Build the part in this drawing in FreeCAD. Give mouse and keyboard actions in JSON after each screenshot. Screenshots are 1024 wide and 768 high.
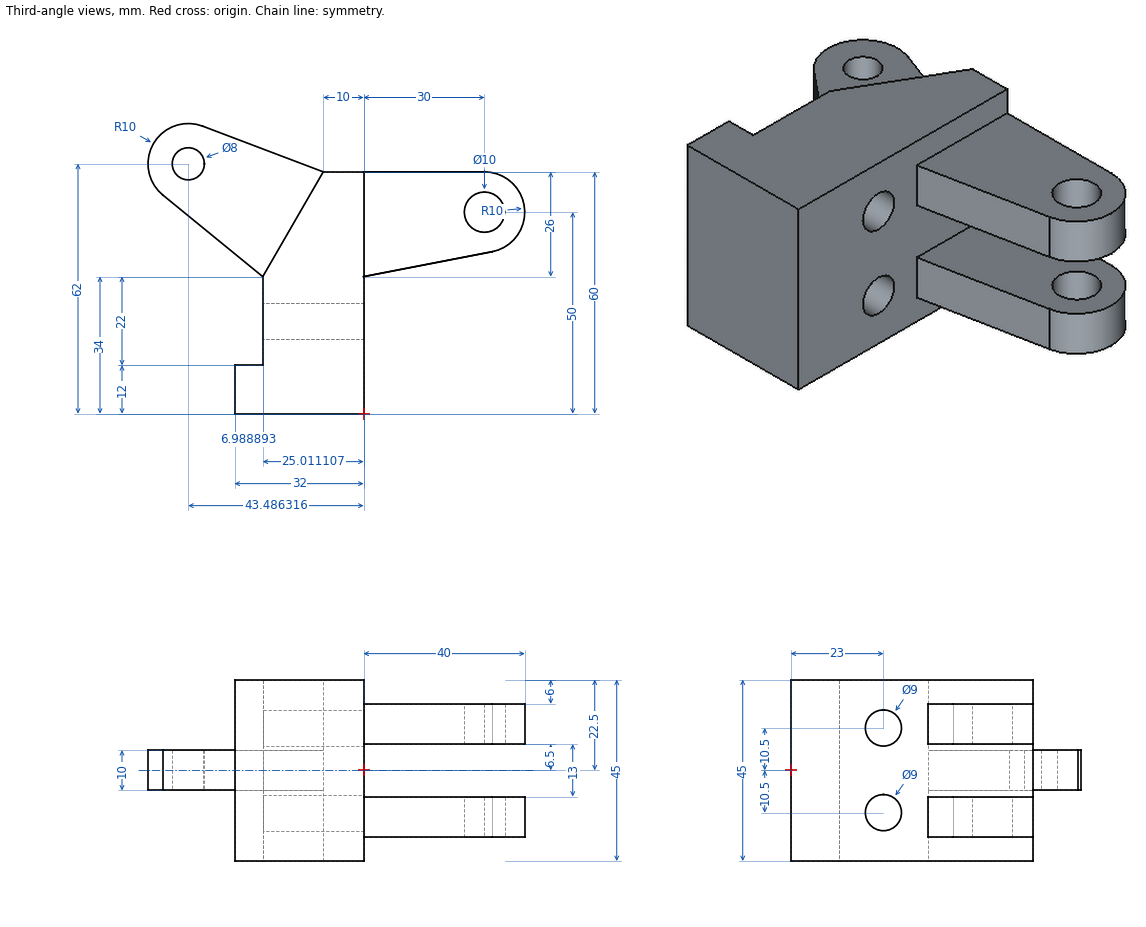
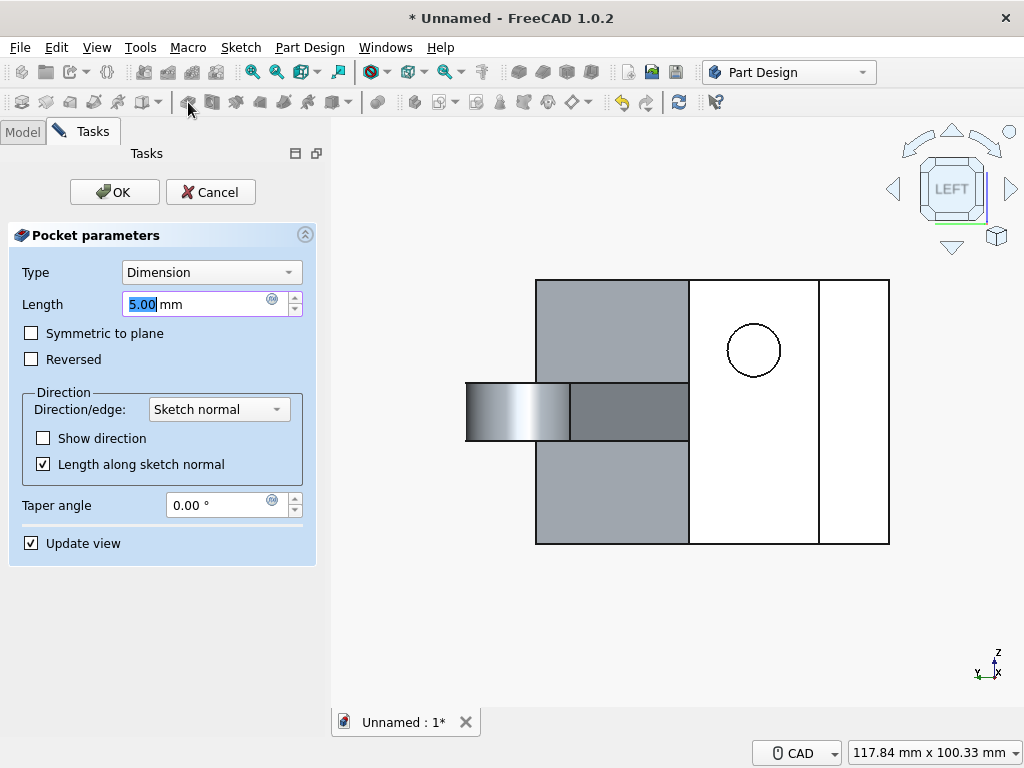
{"action": "left_click", "coordinate": [212, 272]}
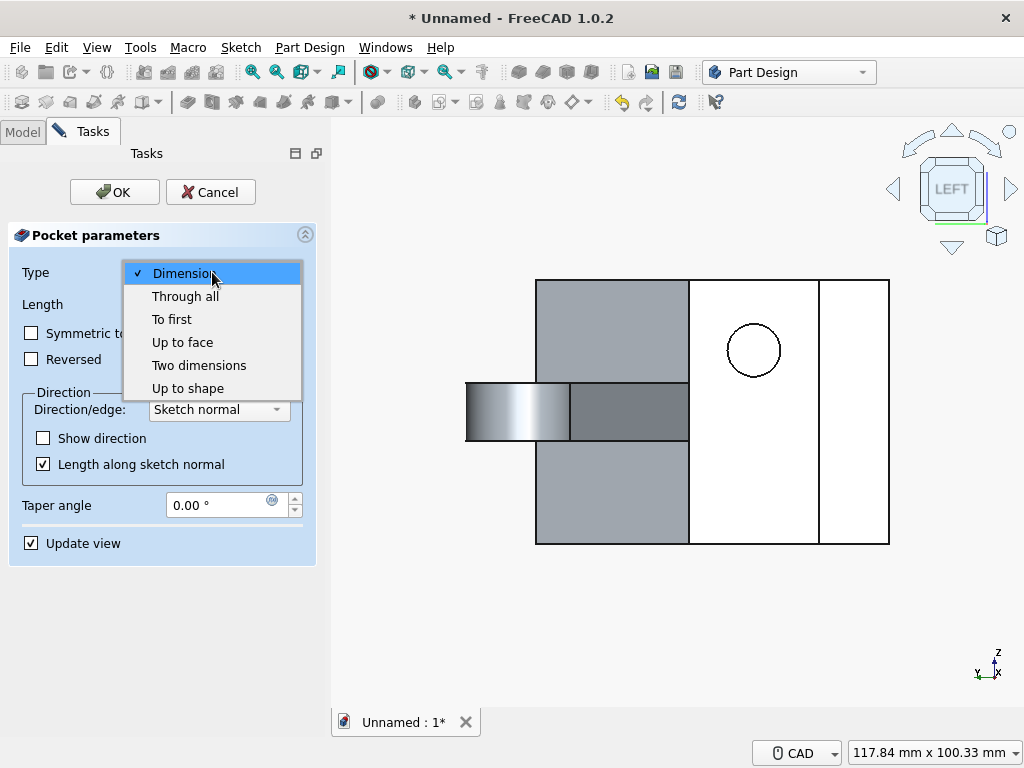
{"action": "left_click", "coordinate": [212, 320]}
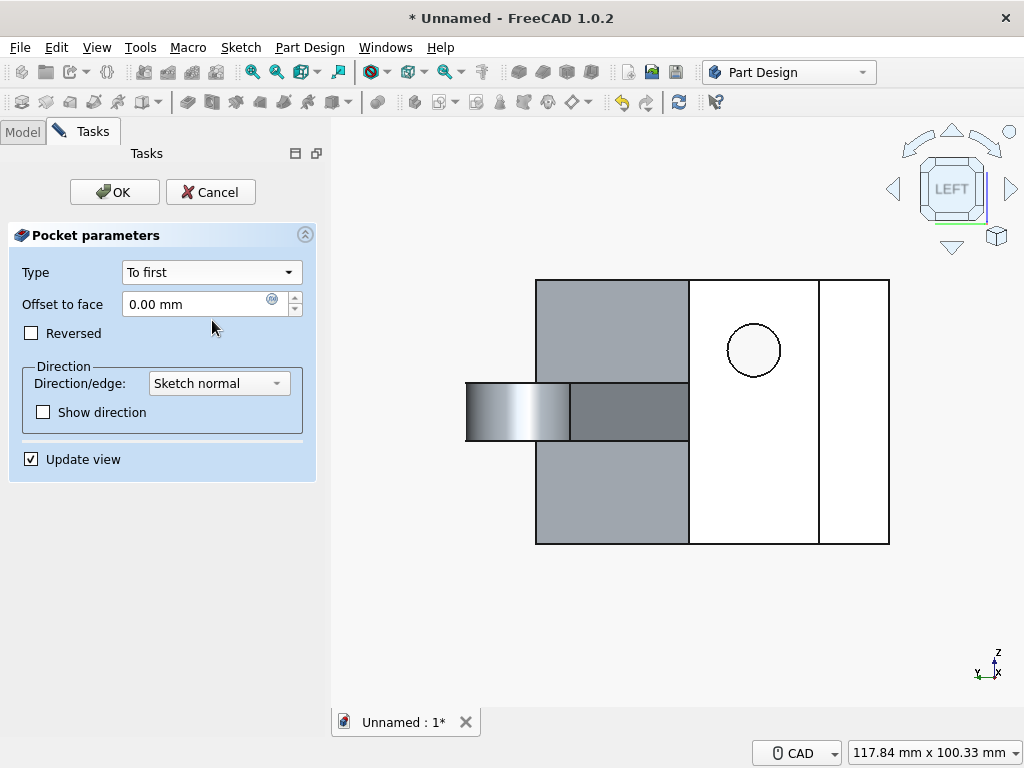
{"action": "left_click", "coordinate": [115, 192]}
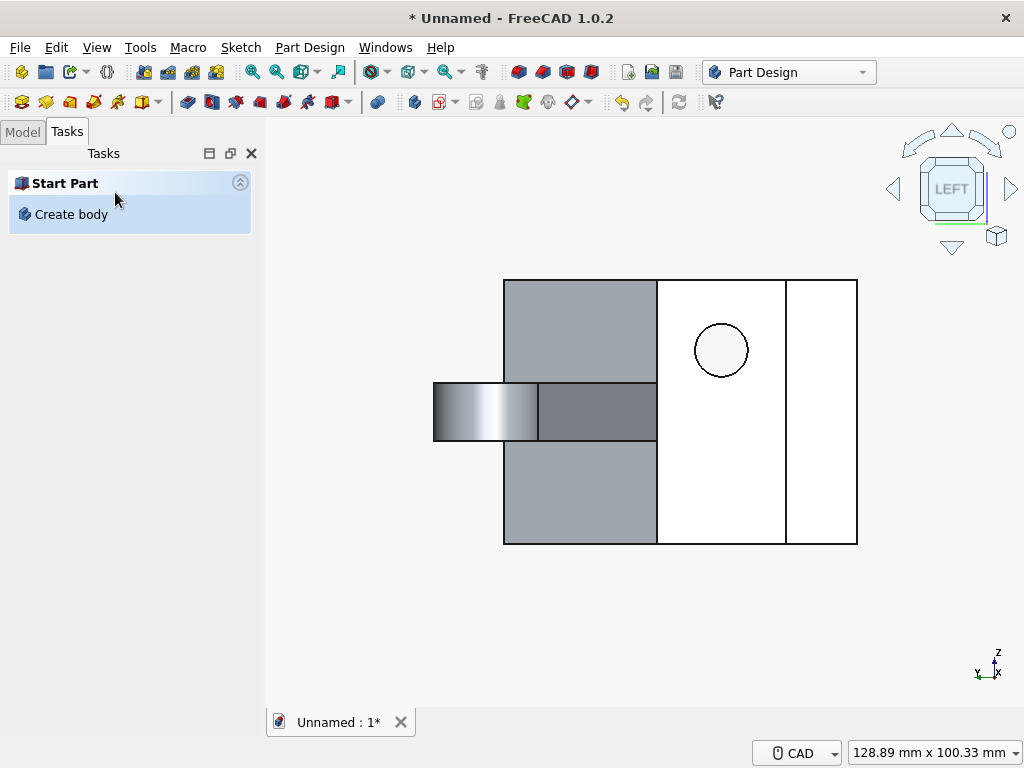
{"action": "left_click", "coordinate": [721, 449]}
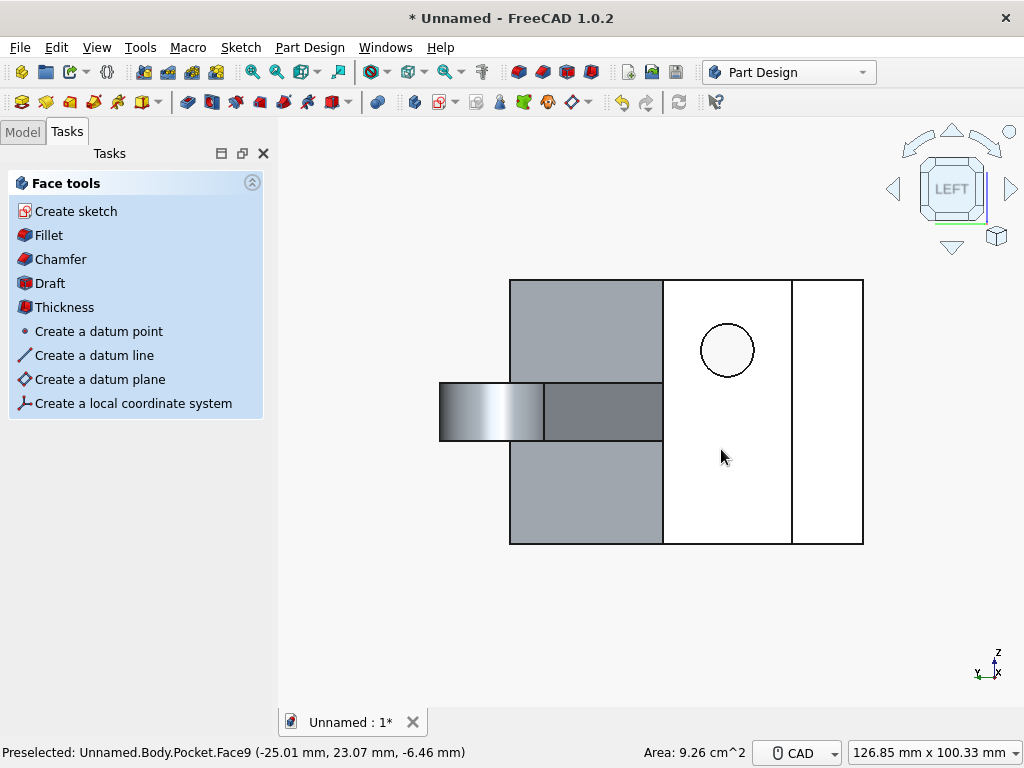
{"action": "left_click", "coordinate": [440, 102]}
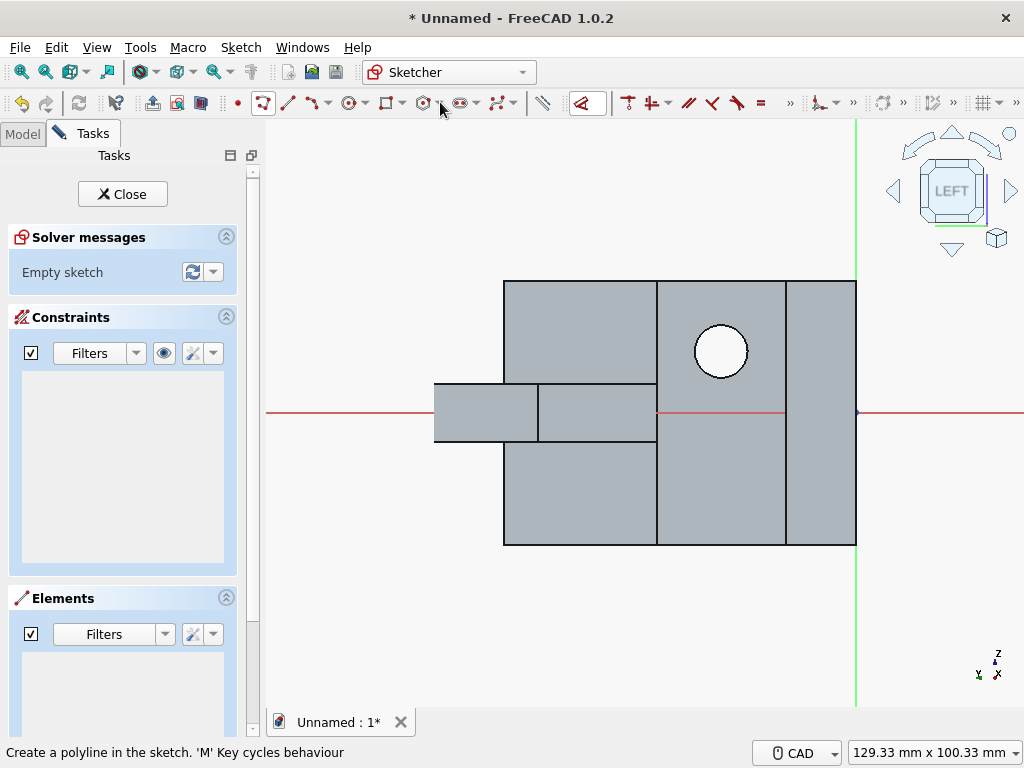
{"action": "key", "text": "q s"}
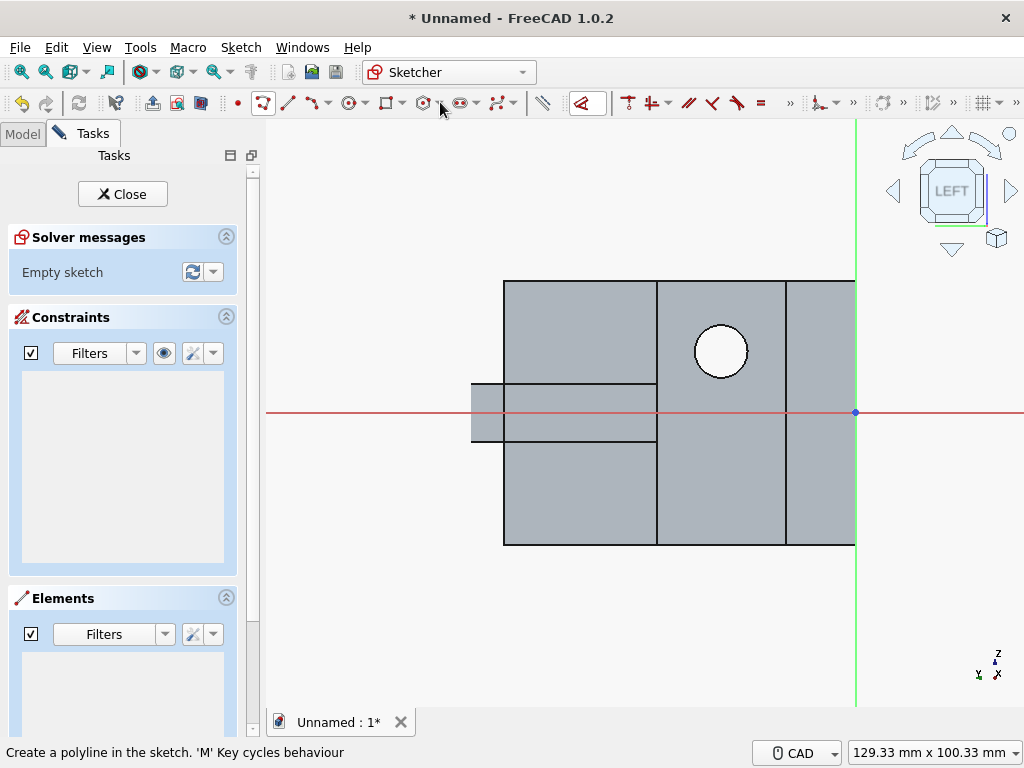
{"action": "scroll", "coordinate": [744, 484], "scroll_direction": "up", "scroll_amount": 10}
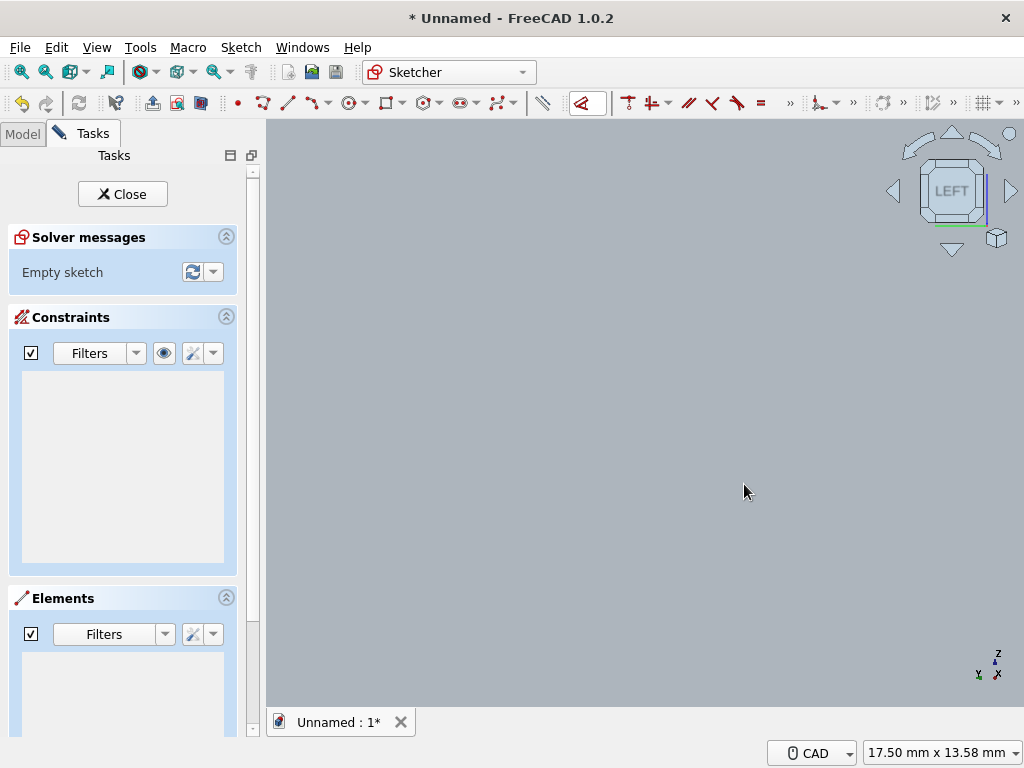
{"action": "key", "text": "g c"}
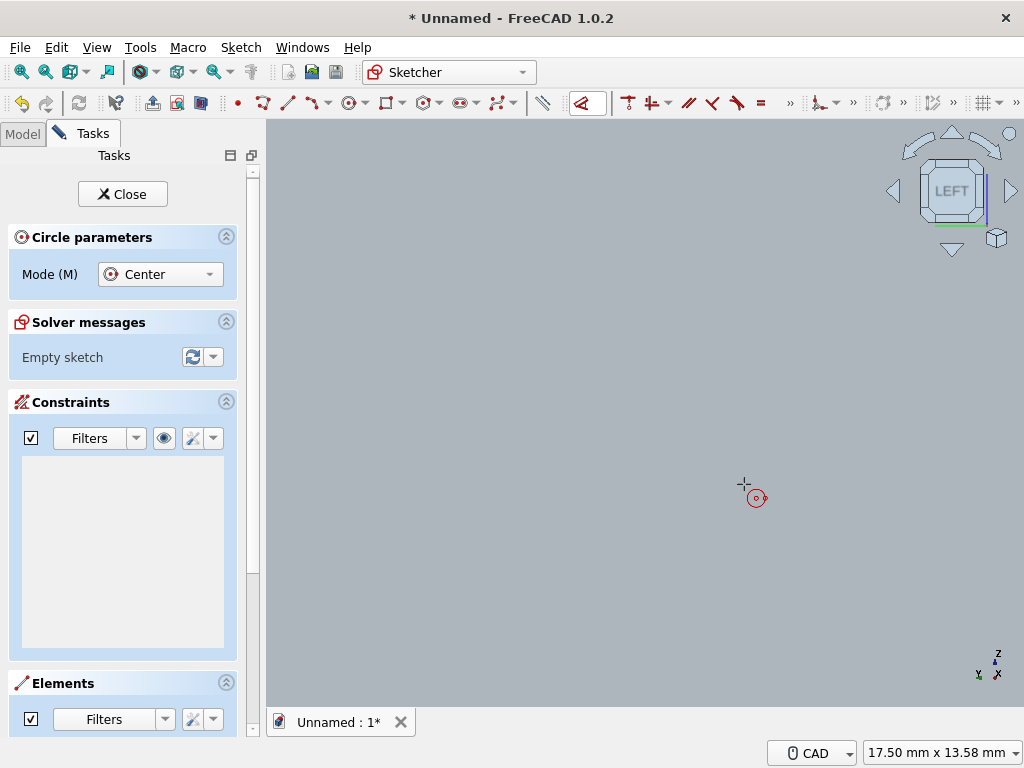
{"action": "left_click", "coordinate": [571, 410]}
{"action": "mouse_move", "coordinate": [709, 272]}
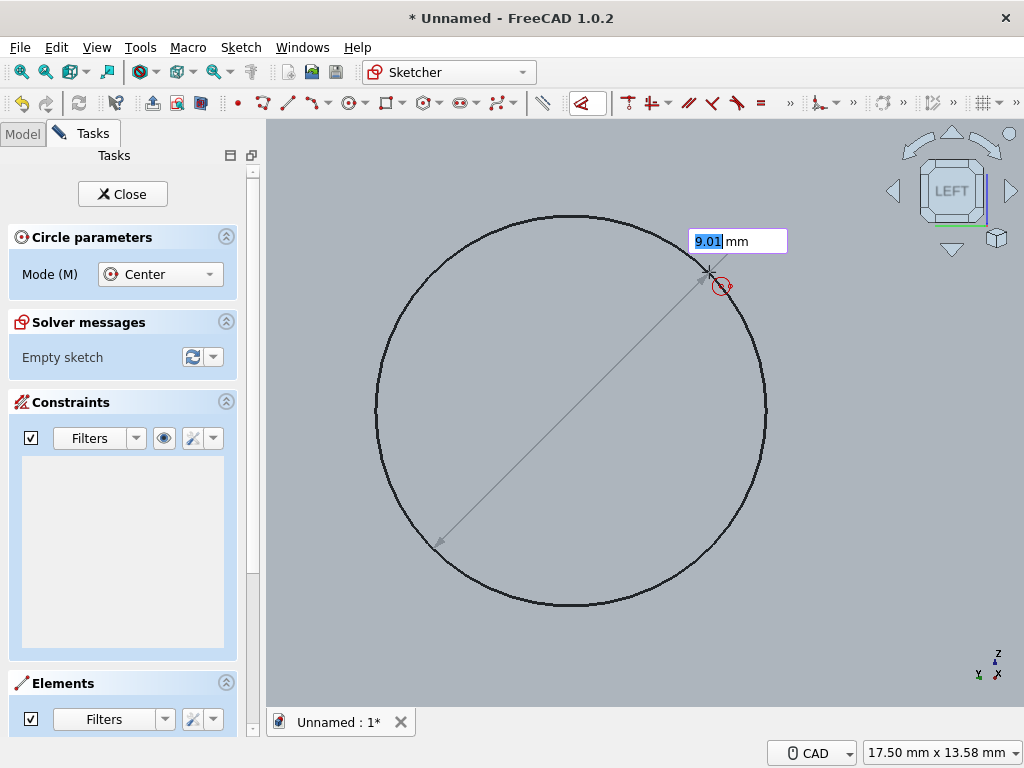
{"action": "type", "text": "9"}
{"action": "key", "text": "Return"}
{"action": "key", "text": "Escape"}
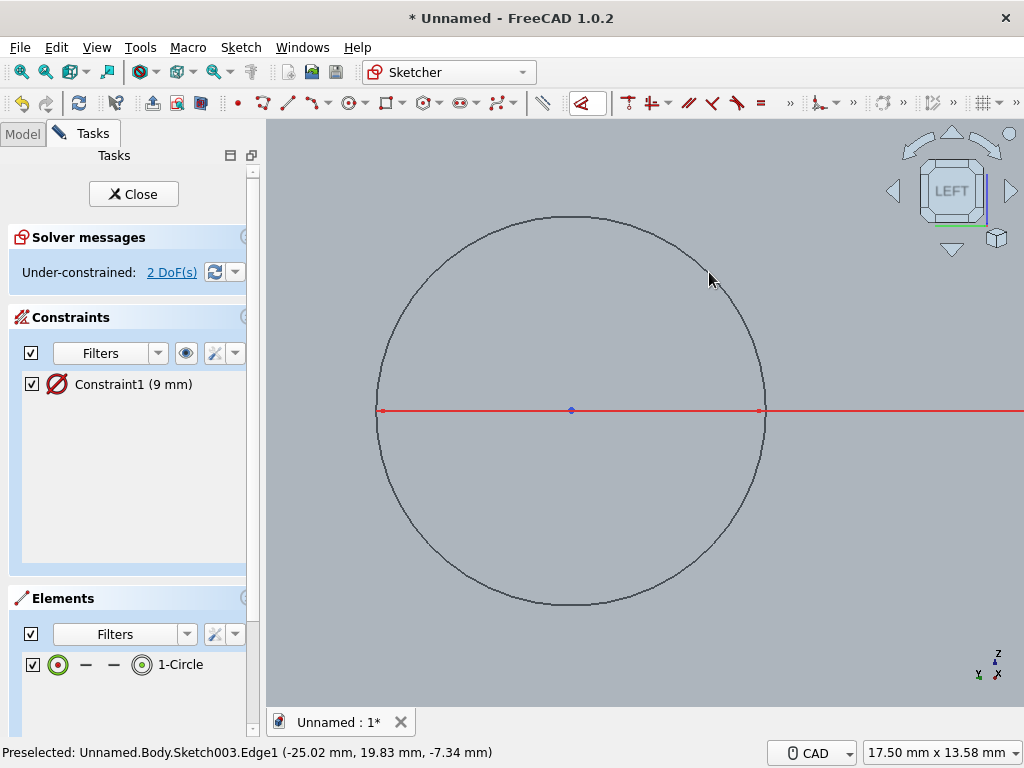
{"action": "left_click", "coordinate": [571, 411]}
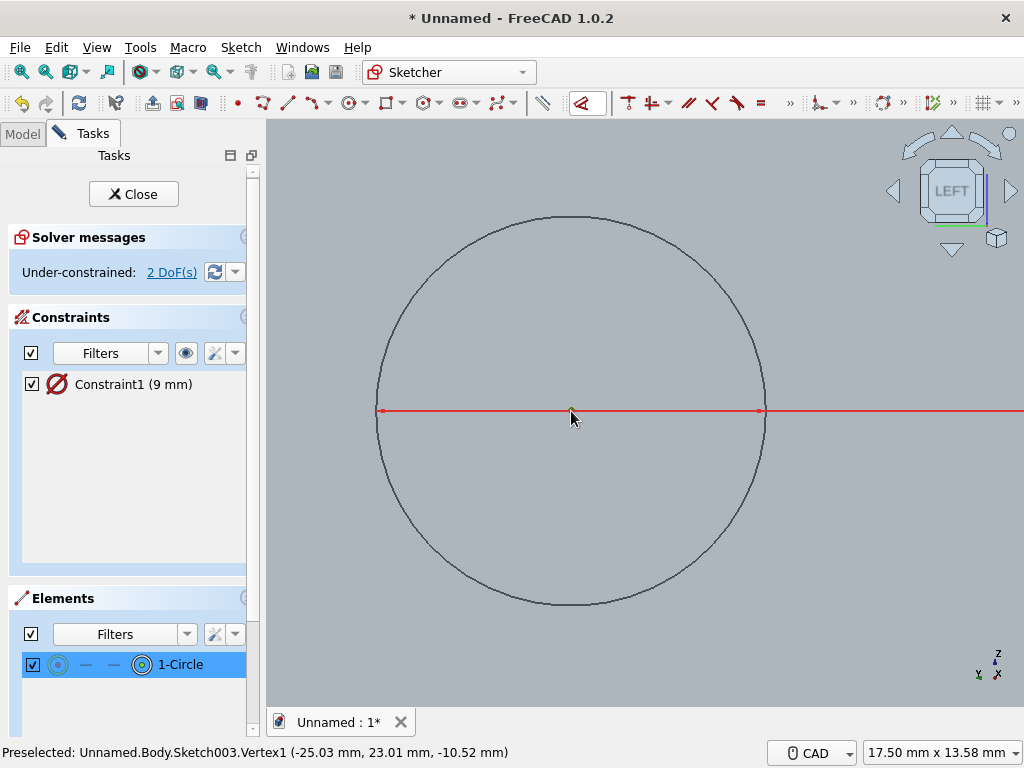
{"action": "left_click", "coordinate": [600, 104]}